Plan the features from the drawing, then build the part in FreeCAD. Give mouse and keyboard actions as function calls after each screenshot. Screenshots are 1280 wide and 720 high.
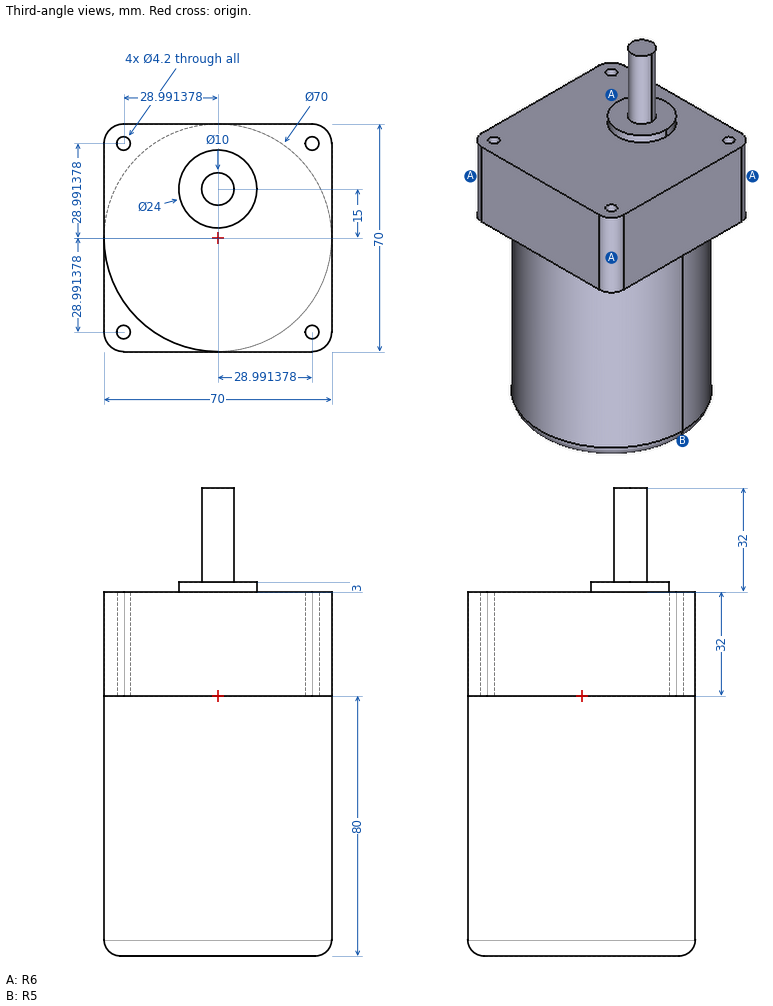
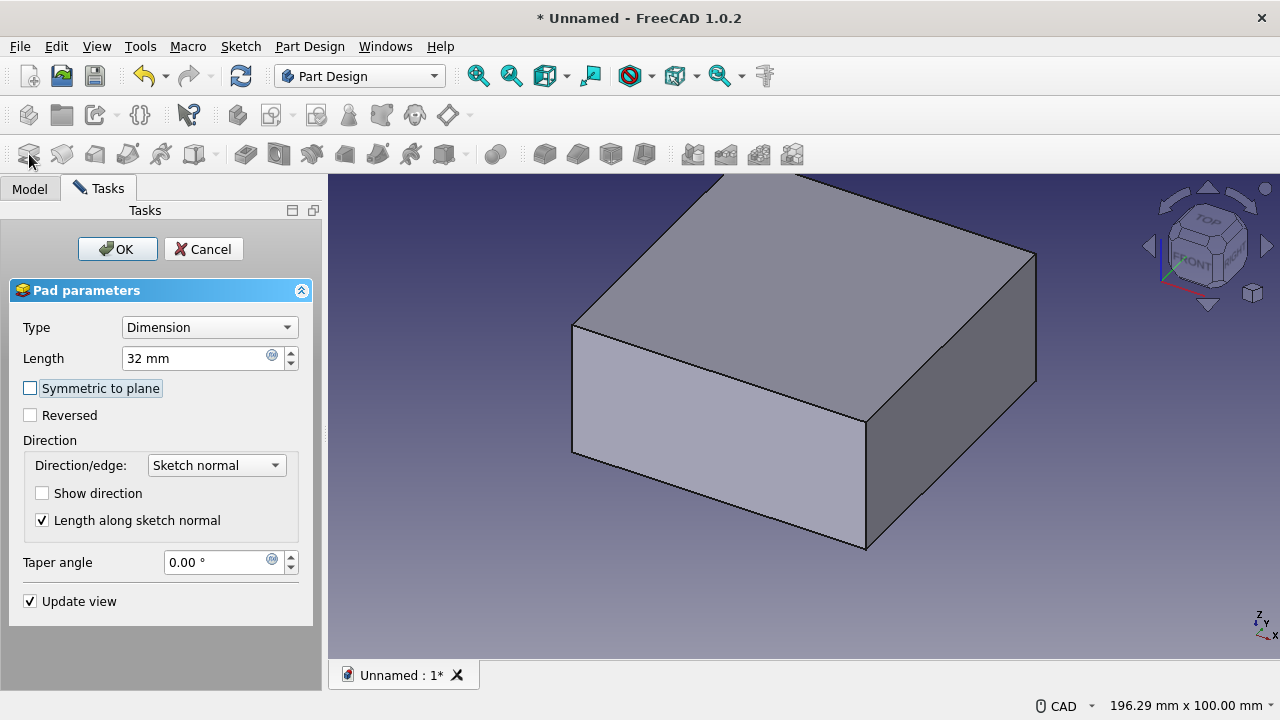
click(118, 249)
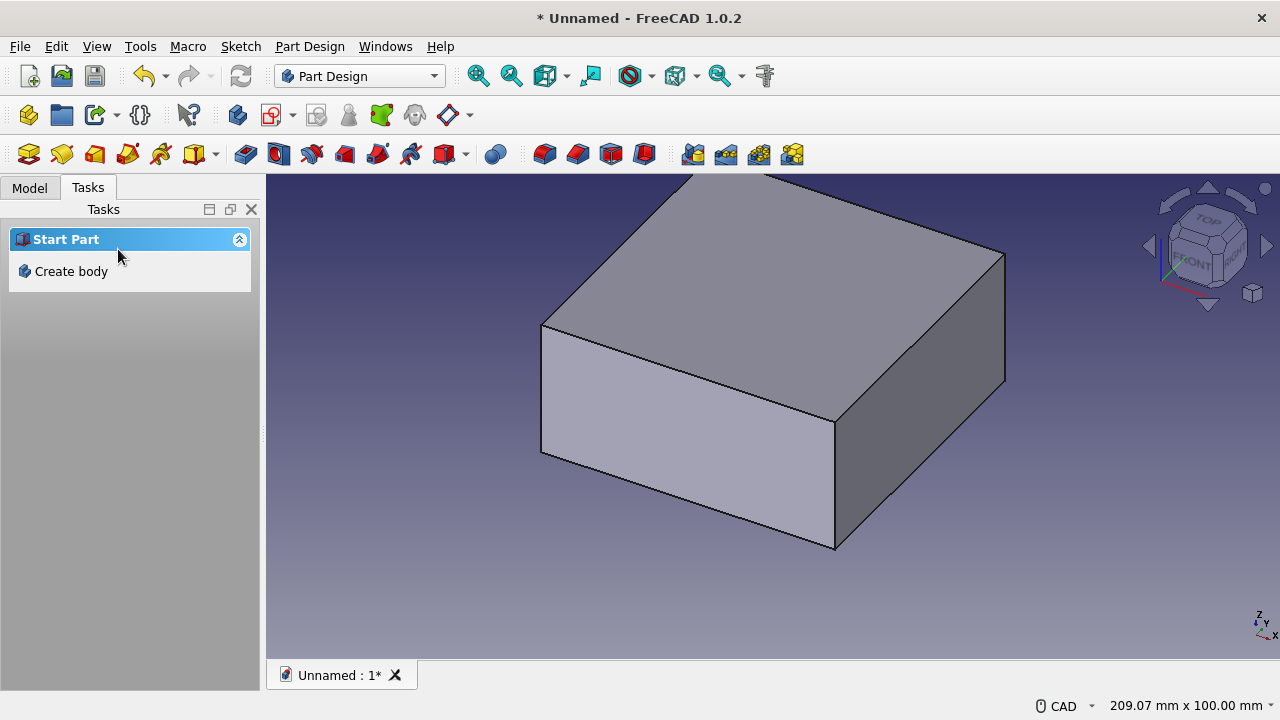
click(479, 76)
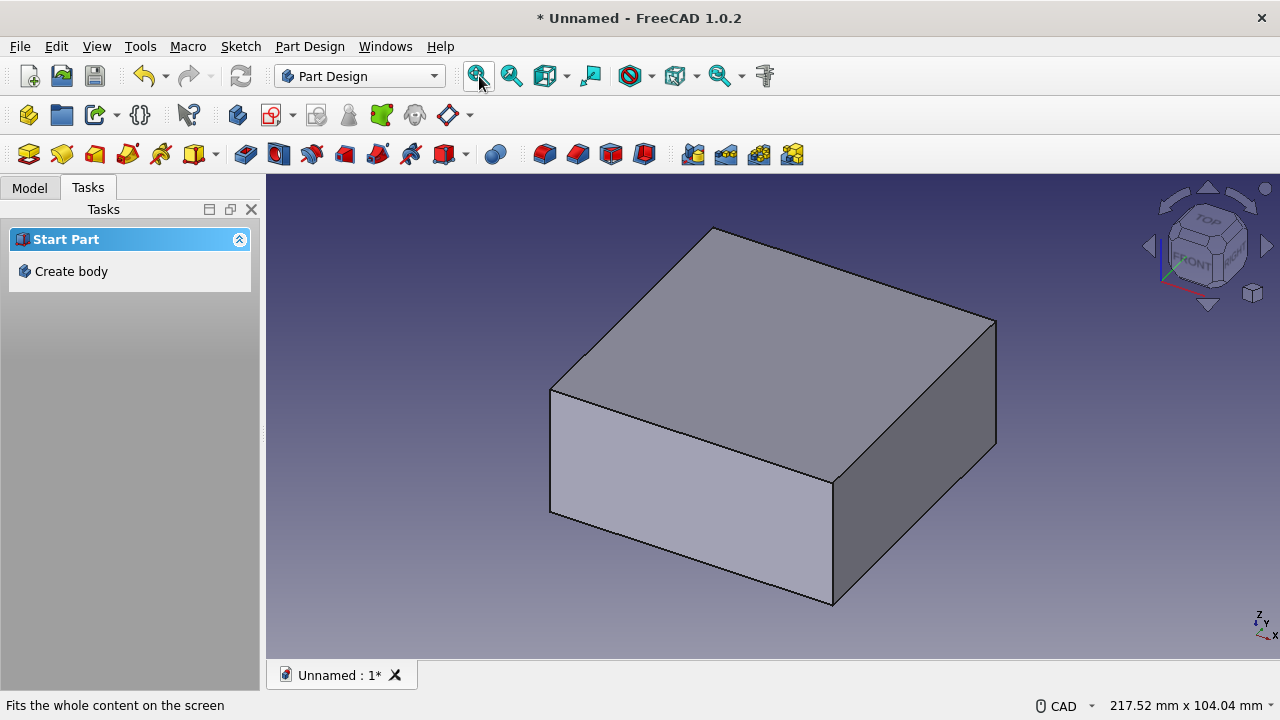
key(5)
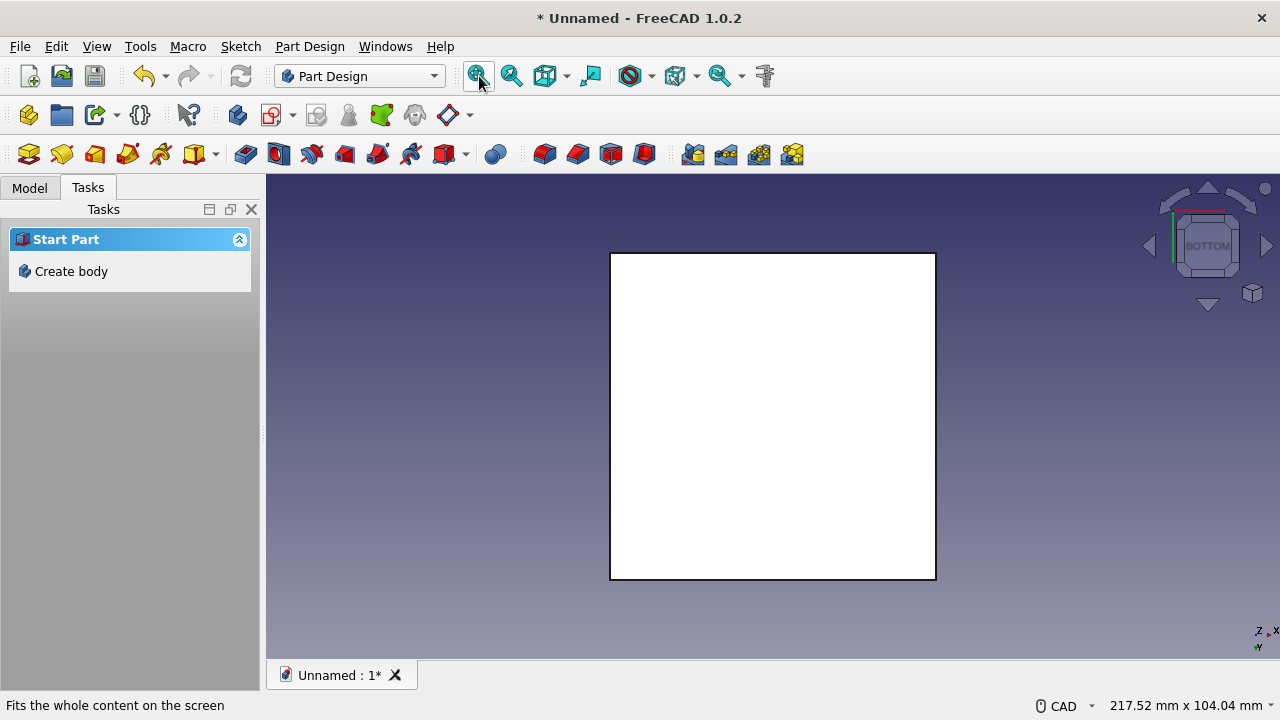
click(773, 415)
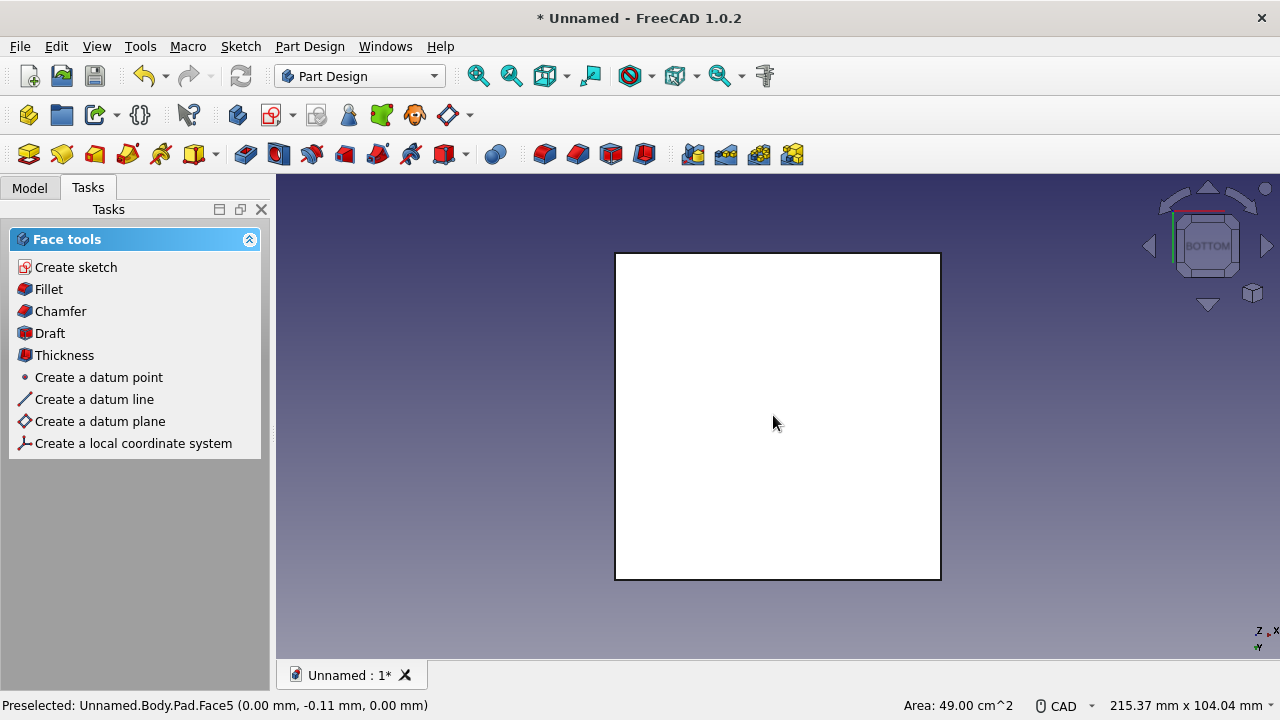
click(270, 116)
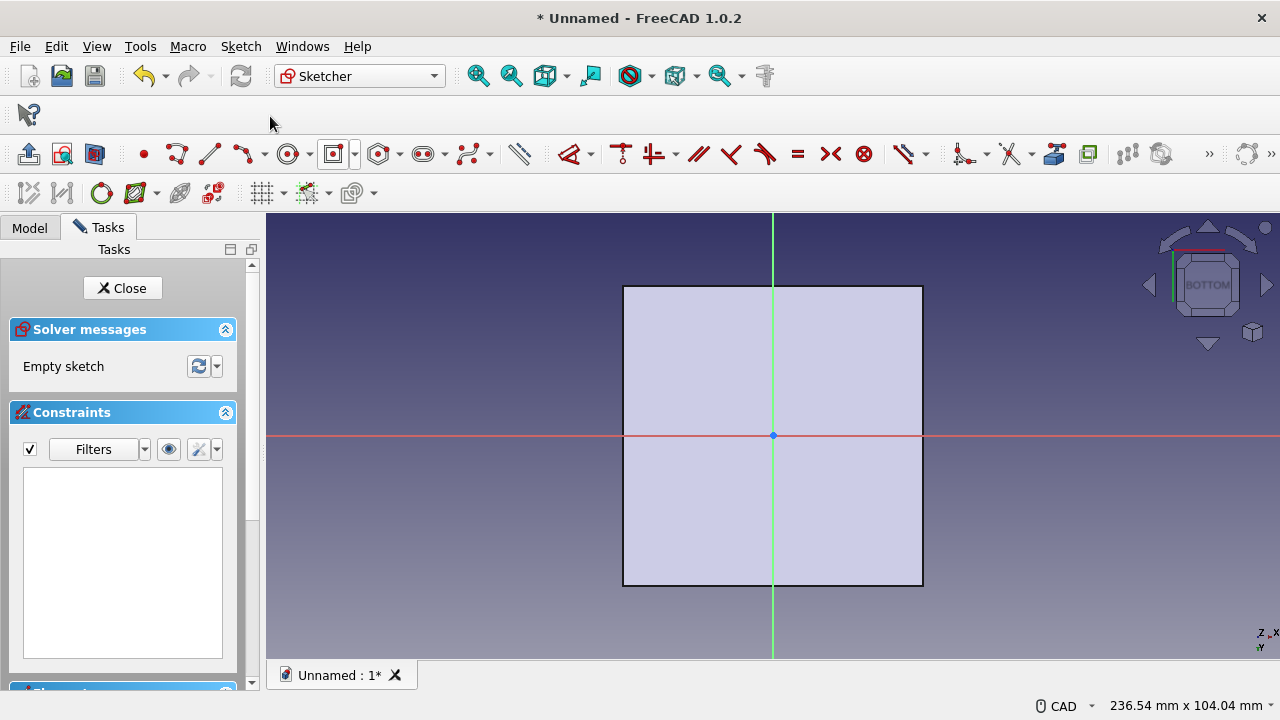
key(g)
key(c)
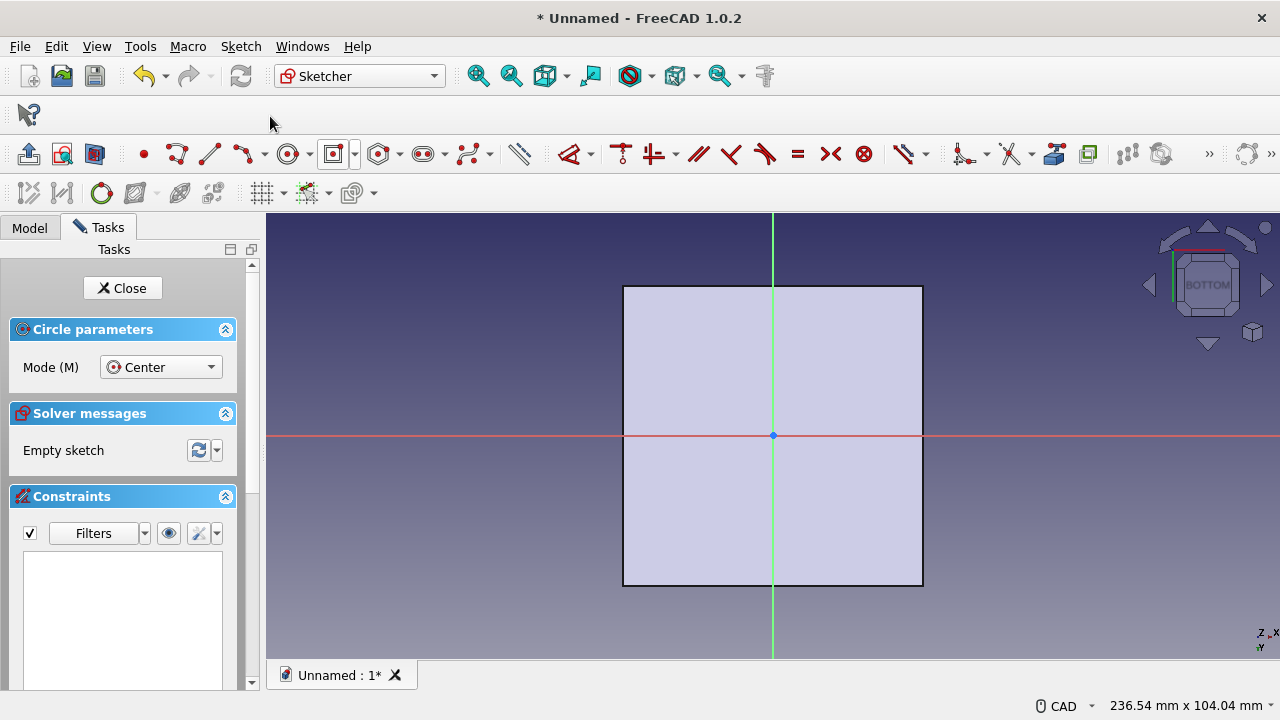
click(773, 436)
move(879, 330)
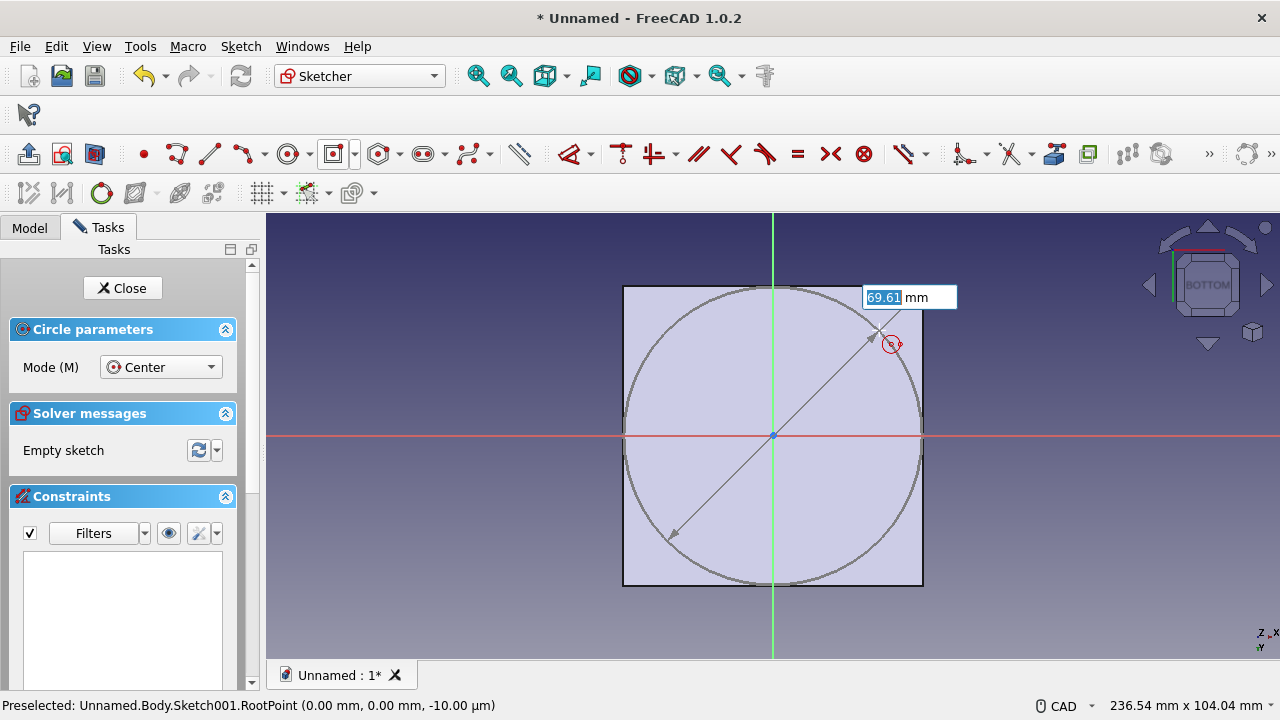
text(70)
key(Return)
key(Escape)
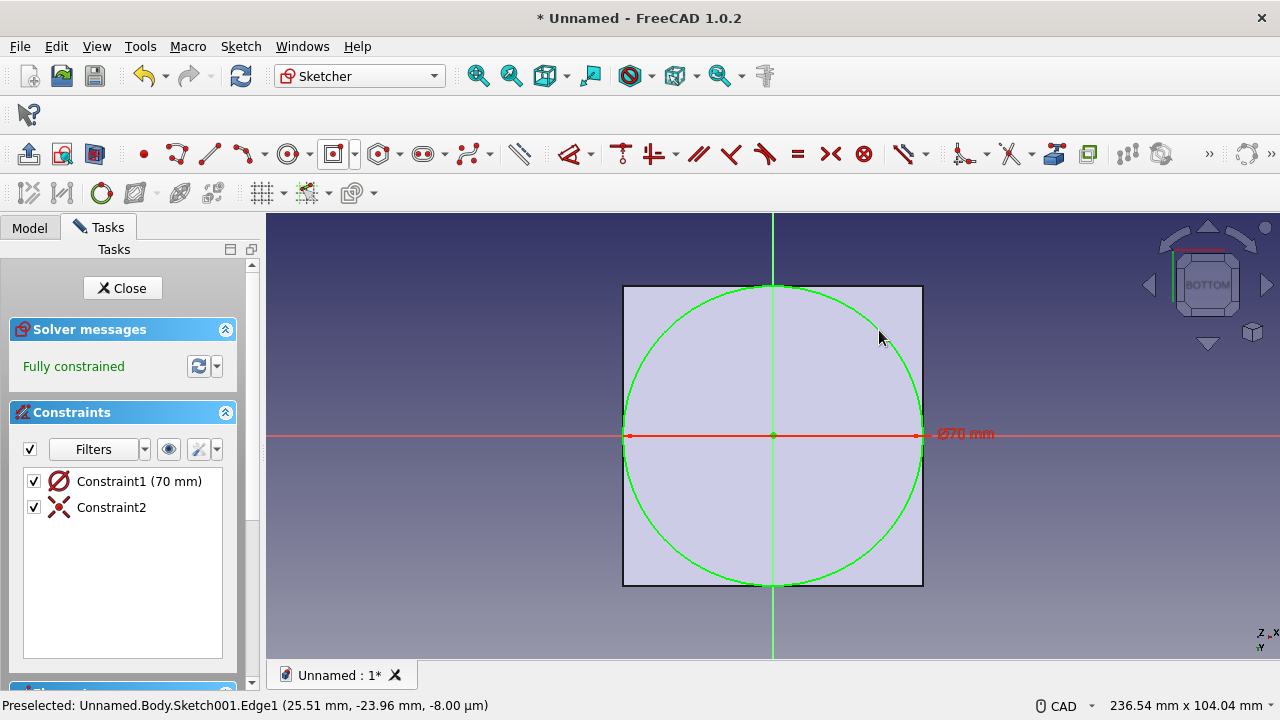
click(123, 288)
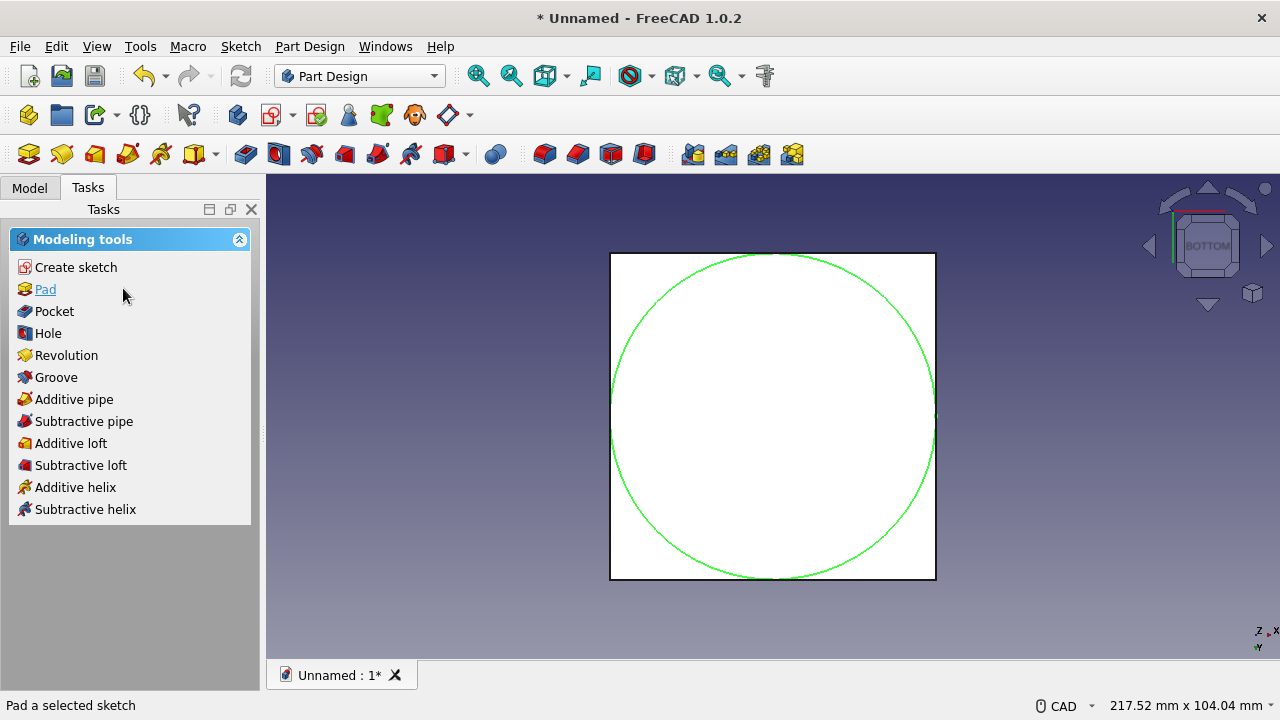
click(29, 154)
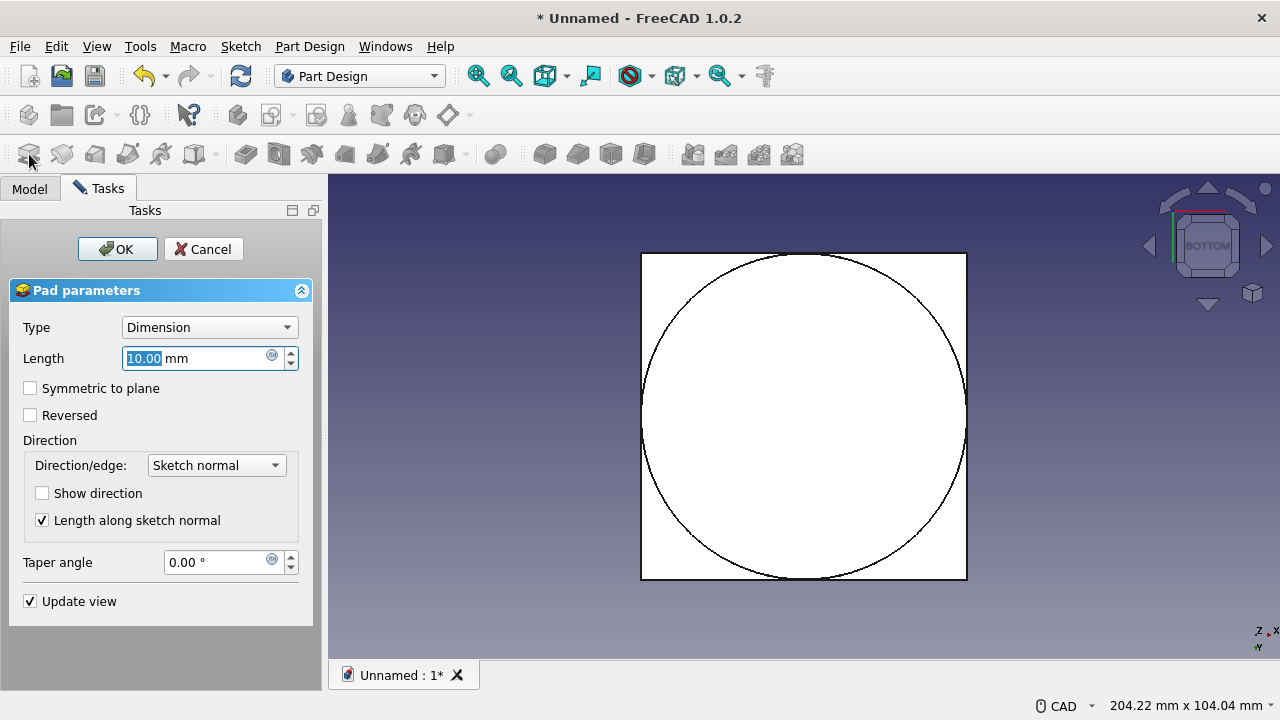
text(80)
key(Tab)